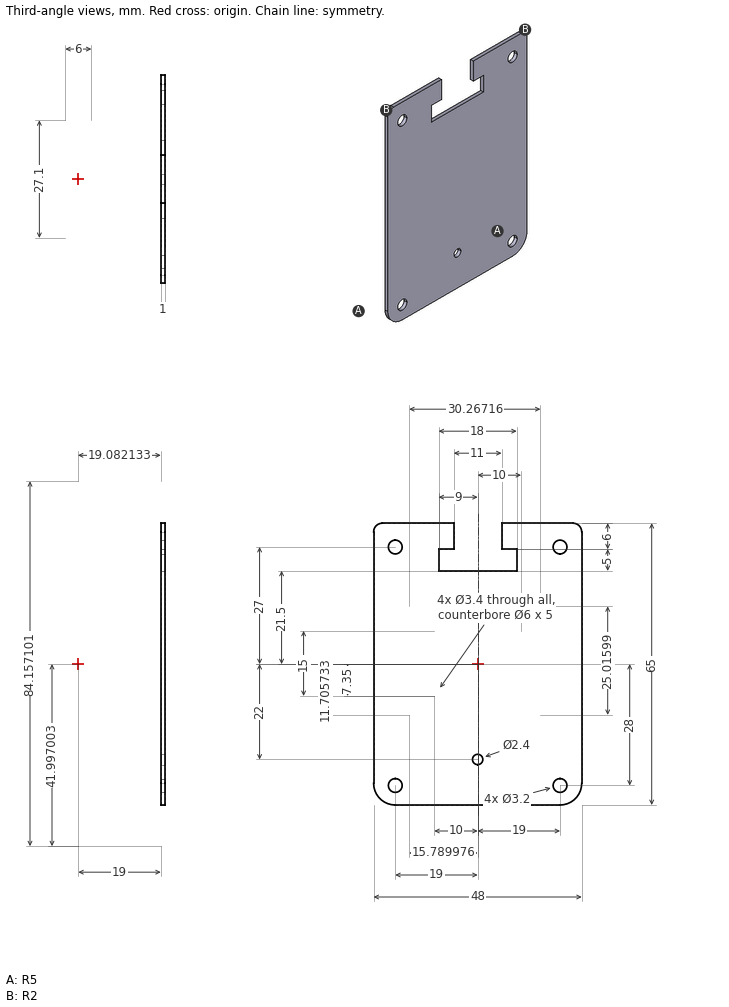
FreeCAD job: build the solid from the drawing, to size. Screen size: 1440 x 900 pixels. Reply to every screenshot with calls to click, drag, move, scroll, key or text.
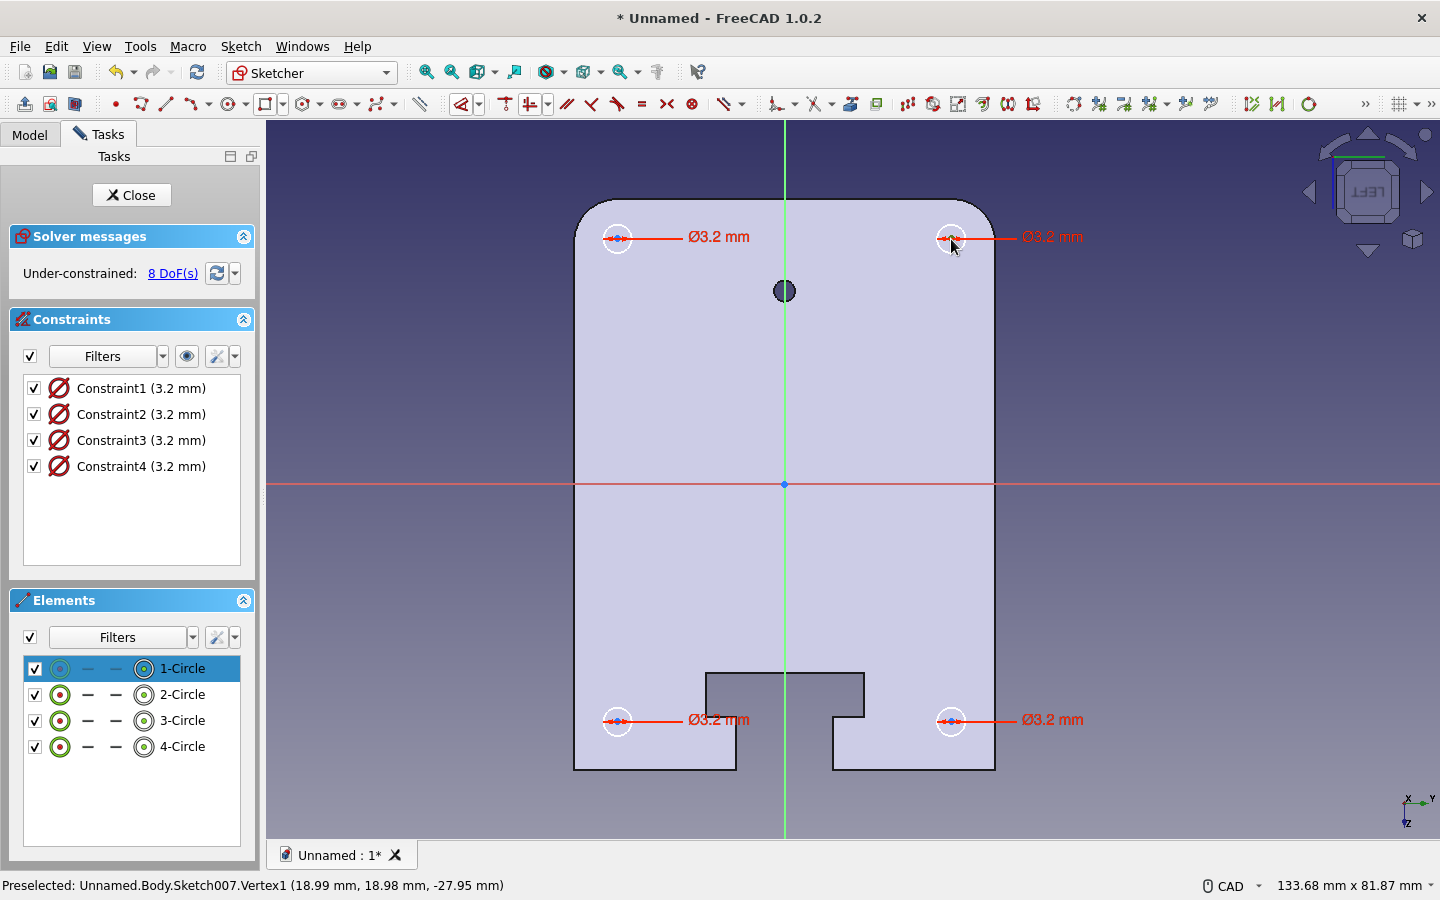
click(618, 239)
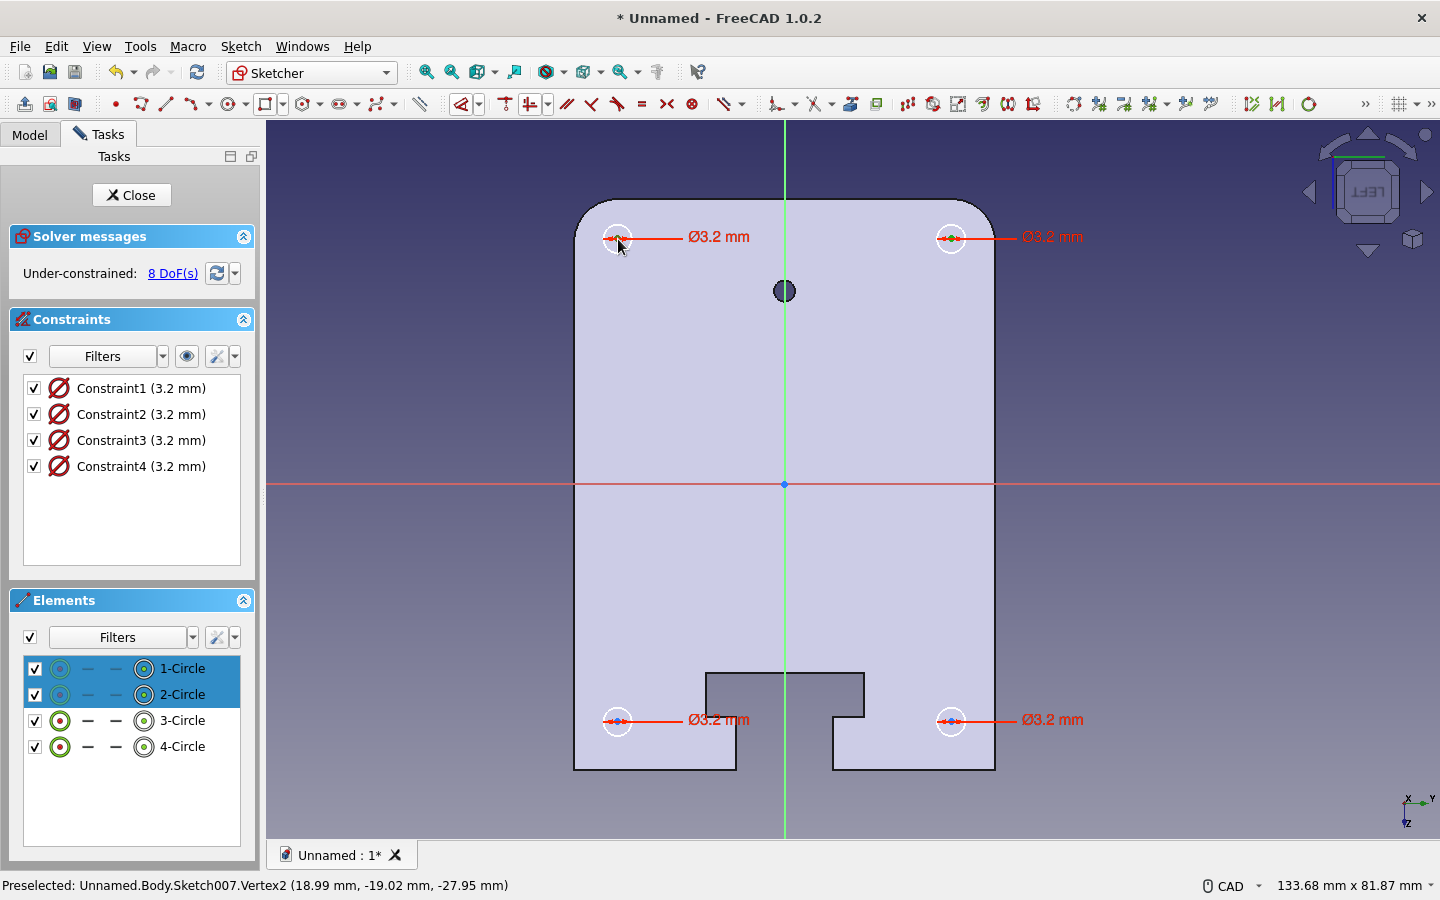
key(h)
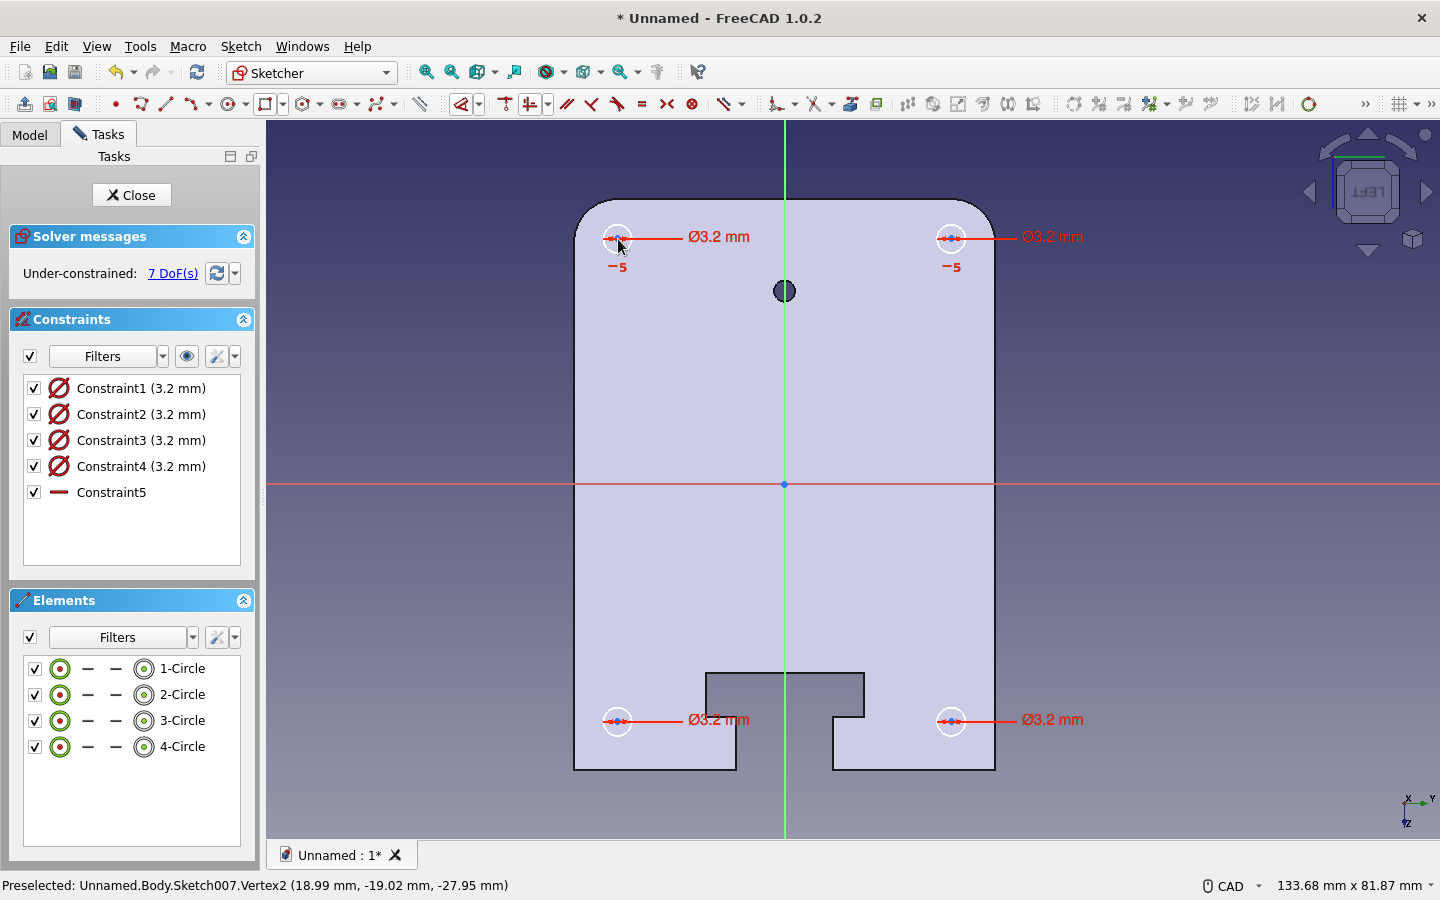
click(618, 239)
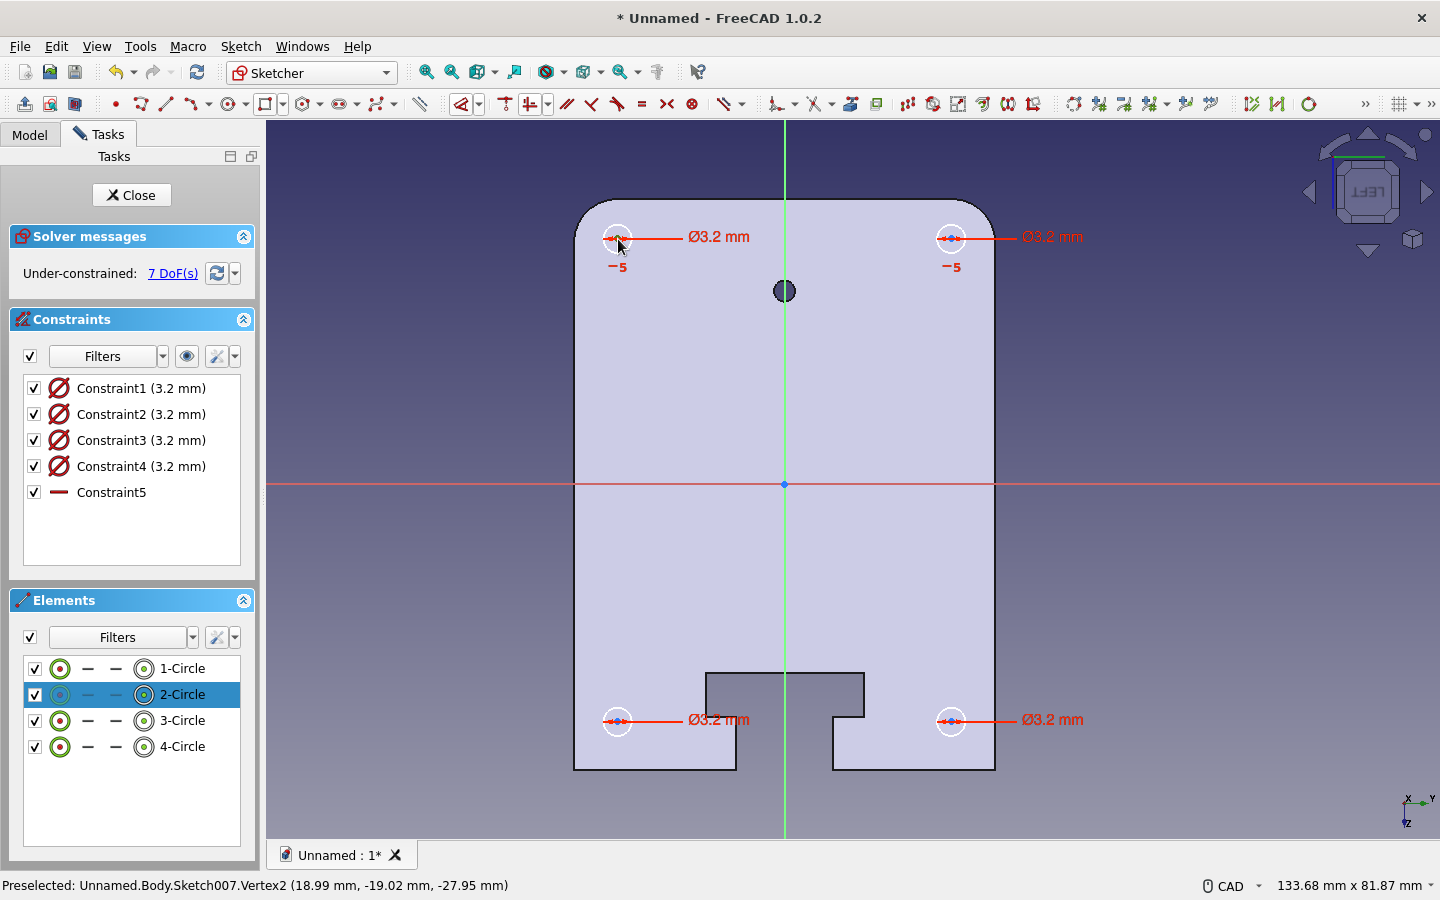
click(618, 722)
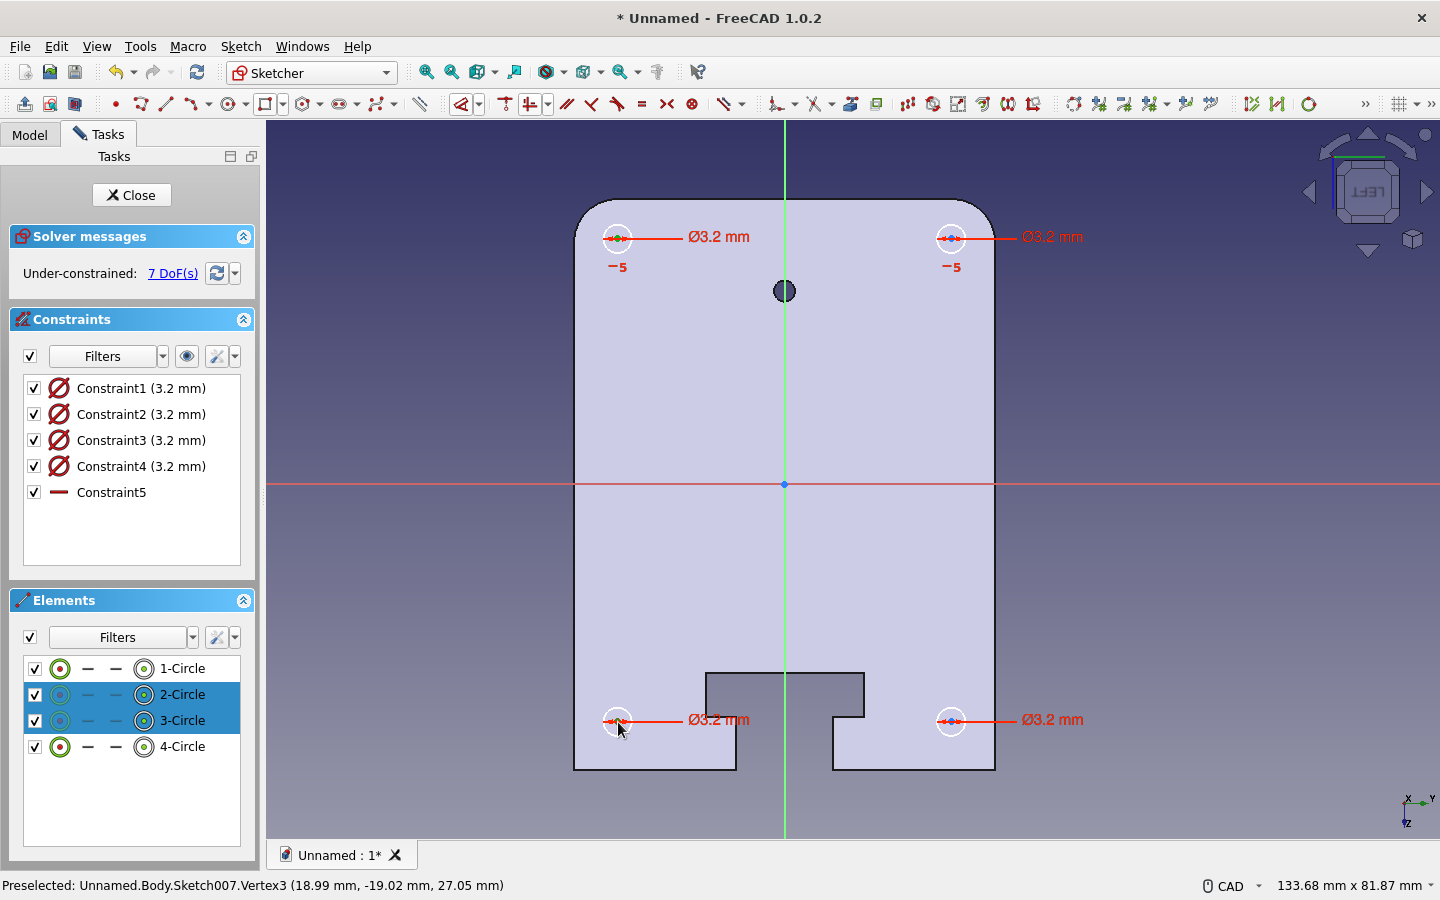
key(v)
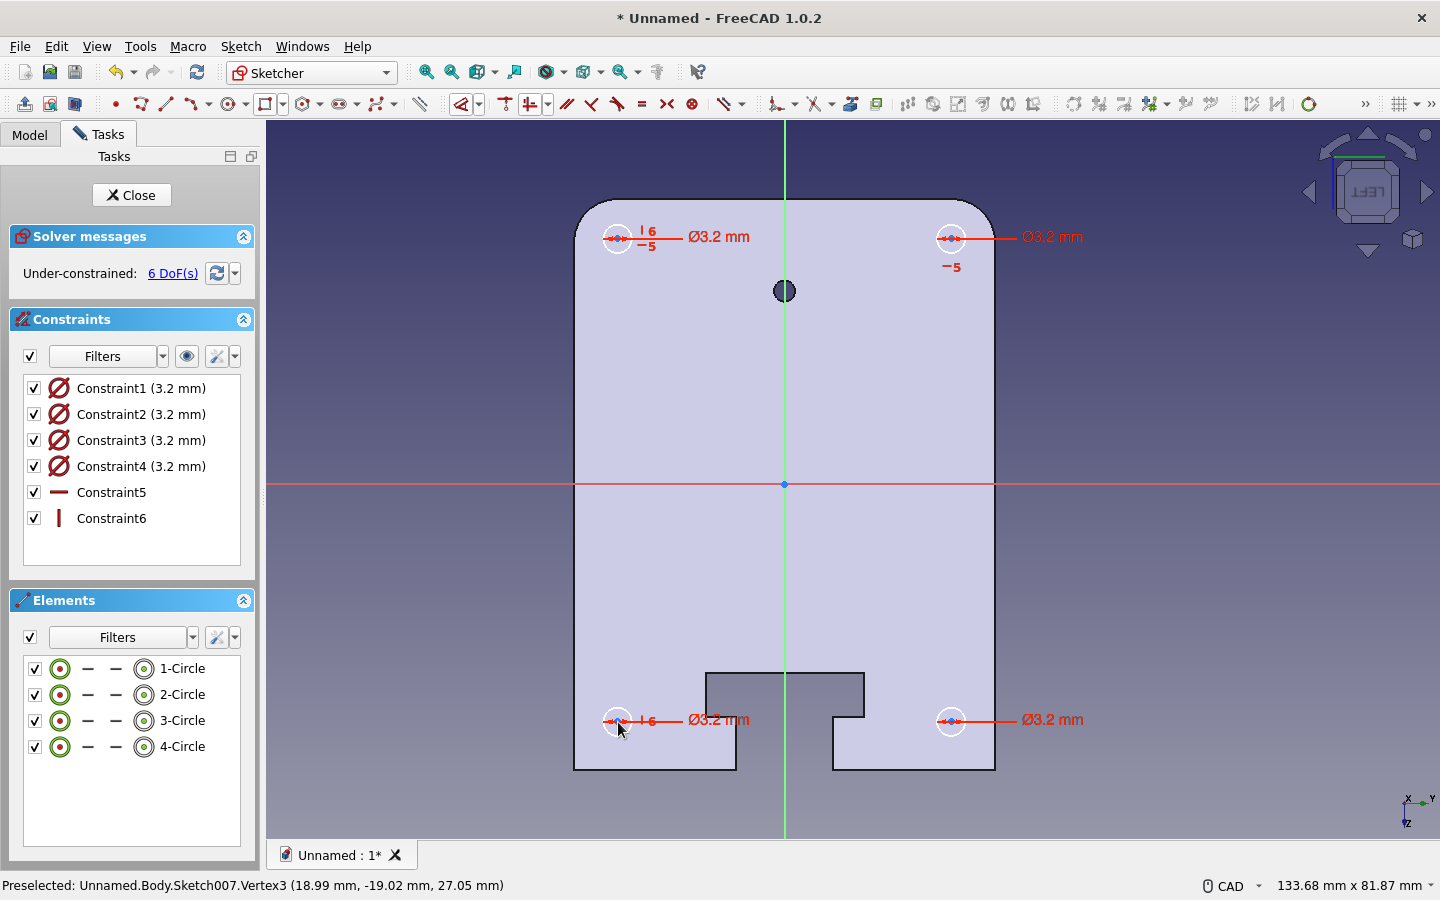
click(951, 239)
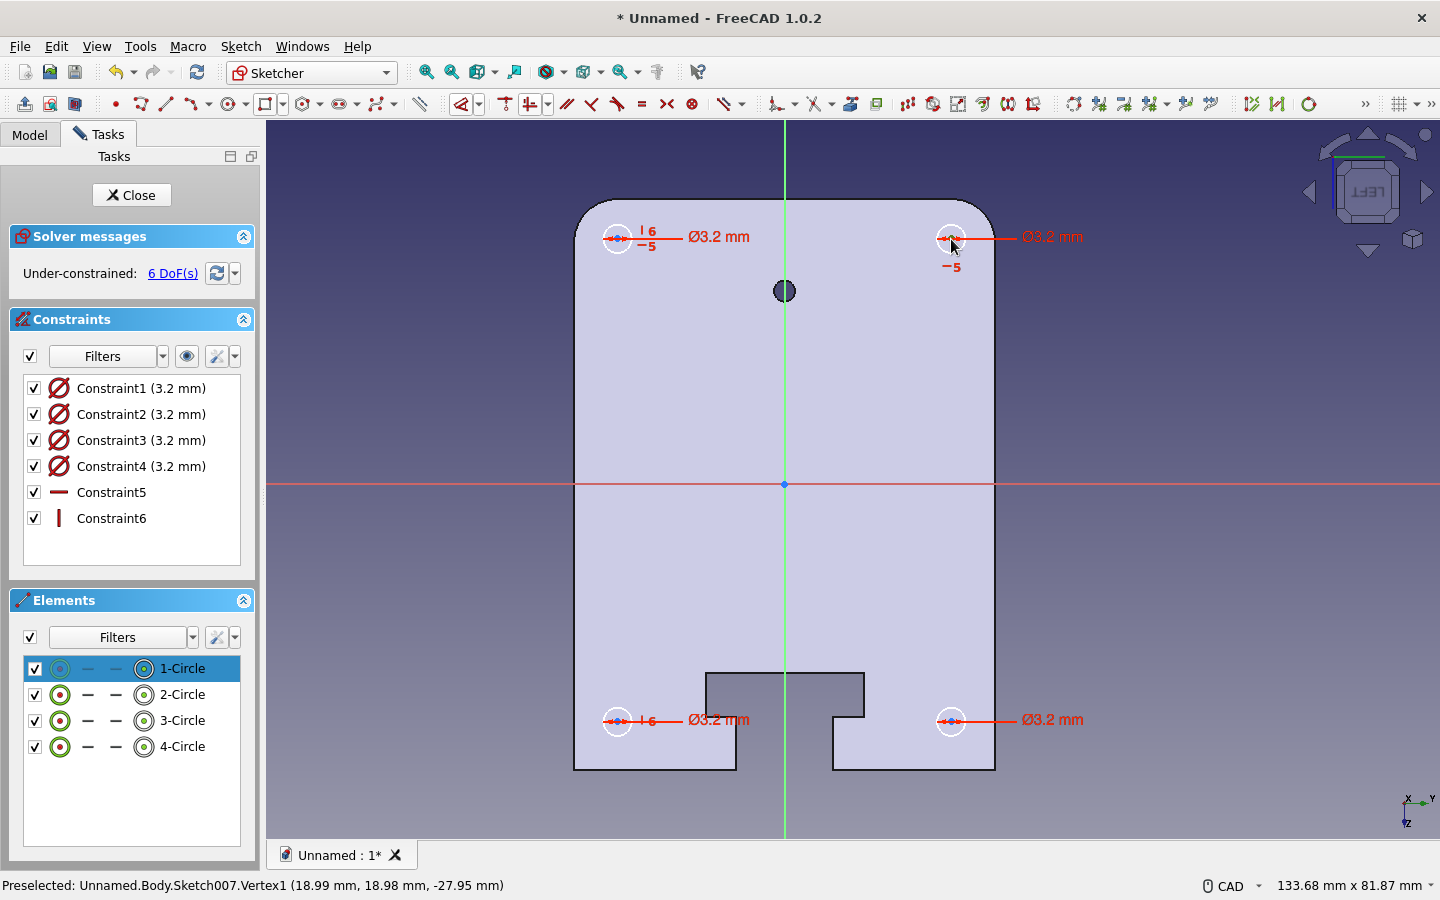
click(951, 722)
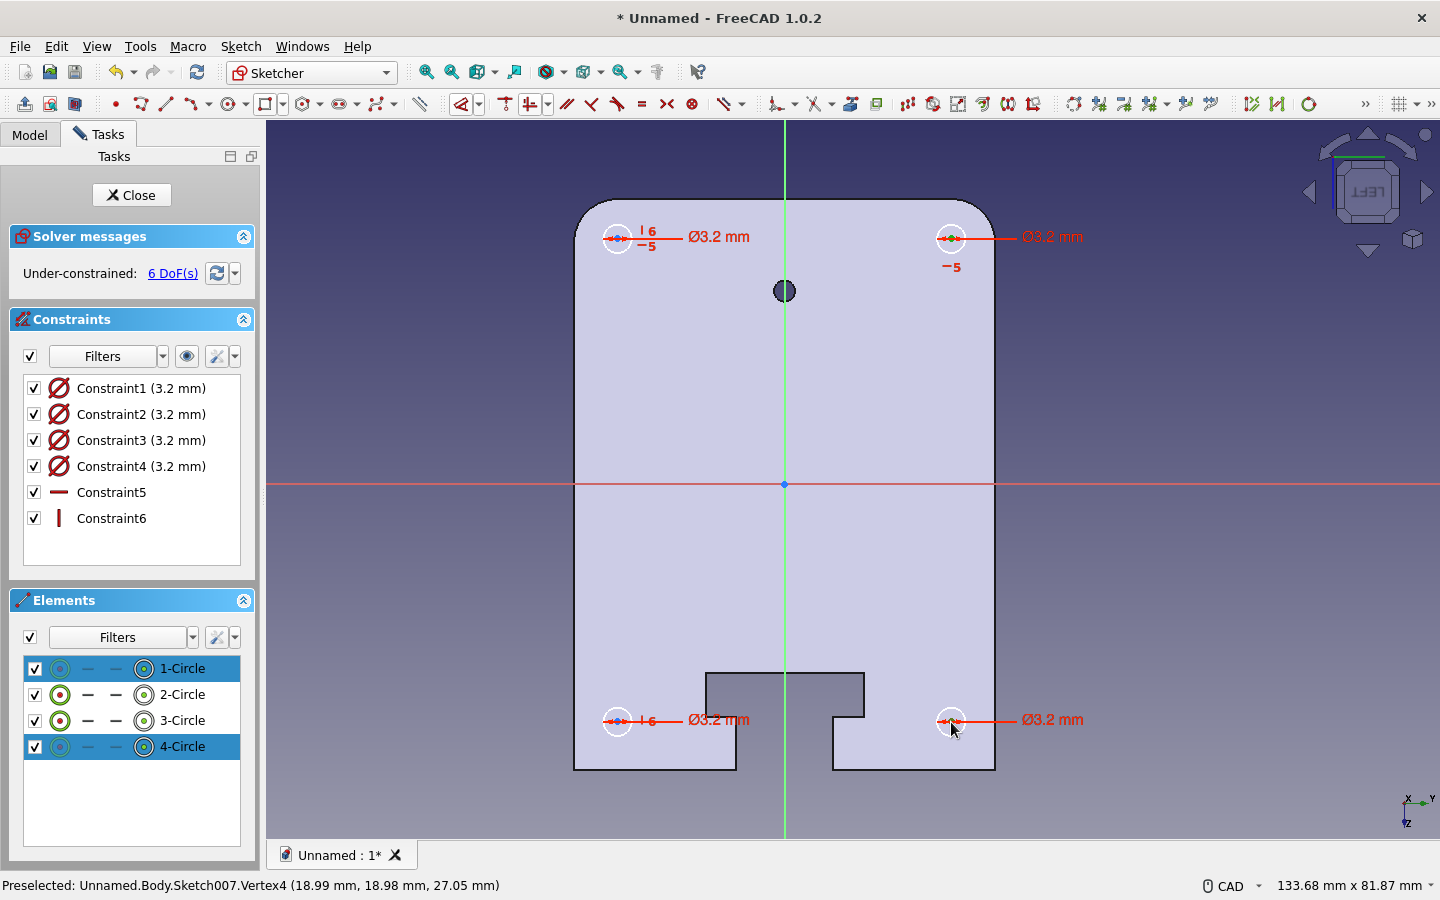
key(v)